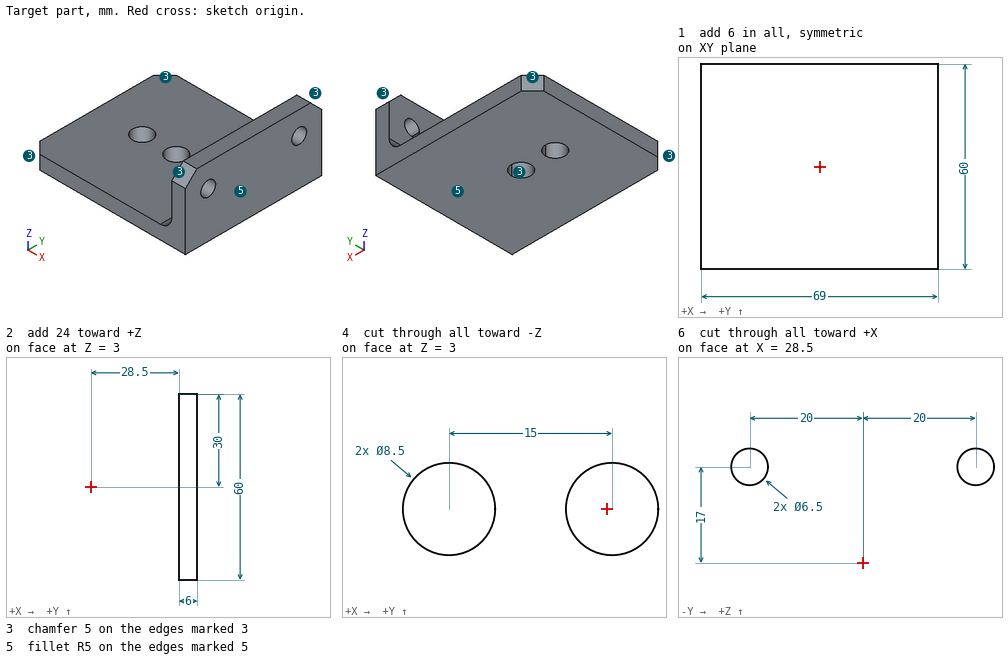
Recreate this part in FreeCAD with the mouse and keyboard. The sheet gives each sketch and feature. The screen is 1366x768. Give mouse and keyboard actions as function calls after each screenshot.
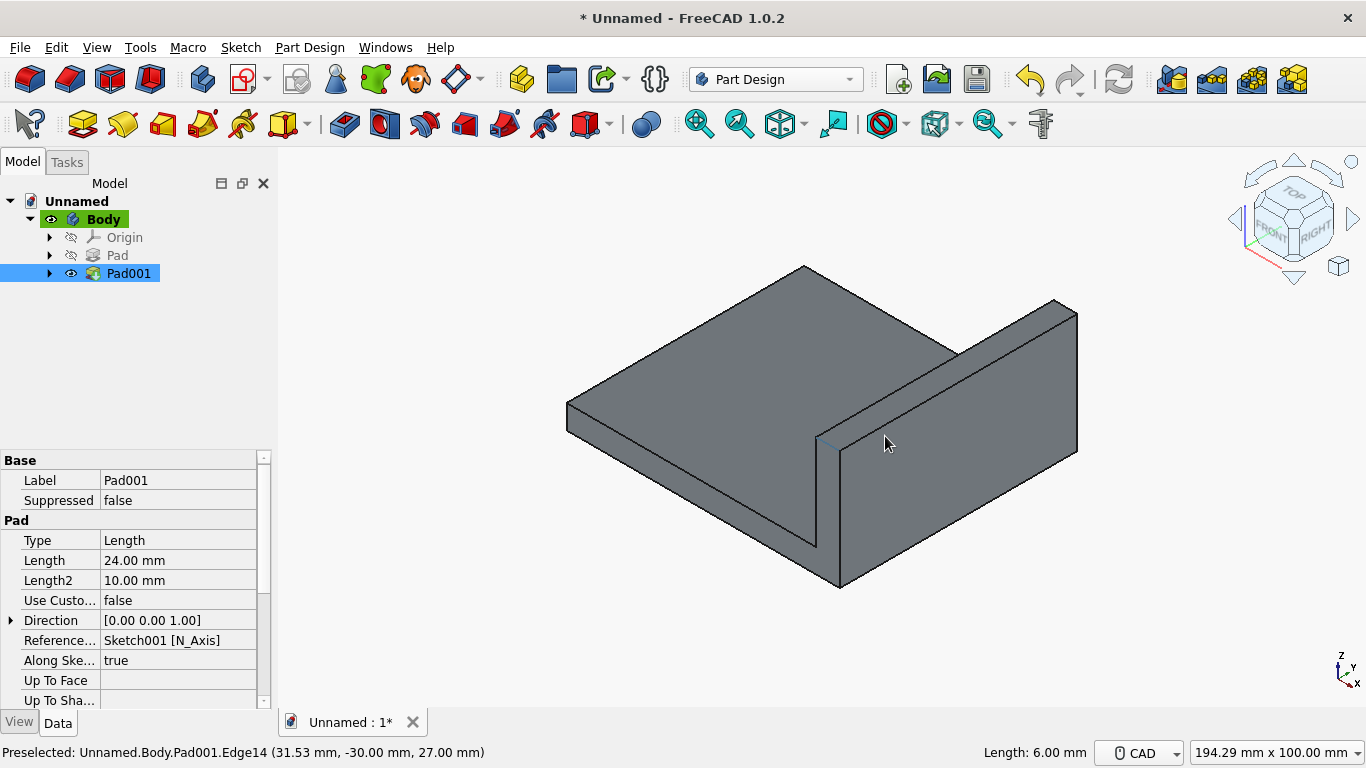
key(2)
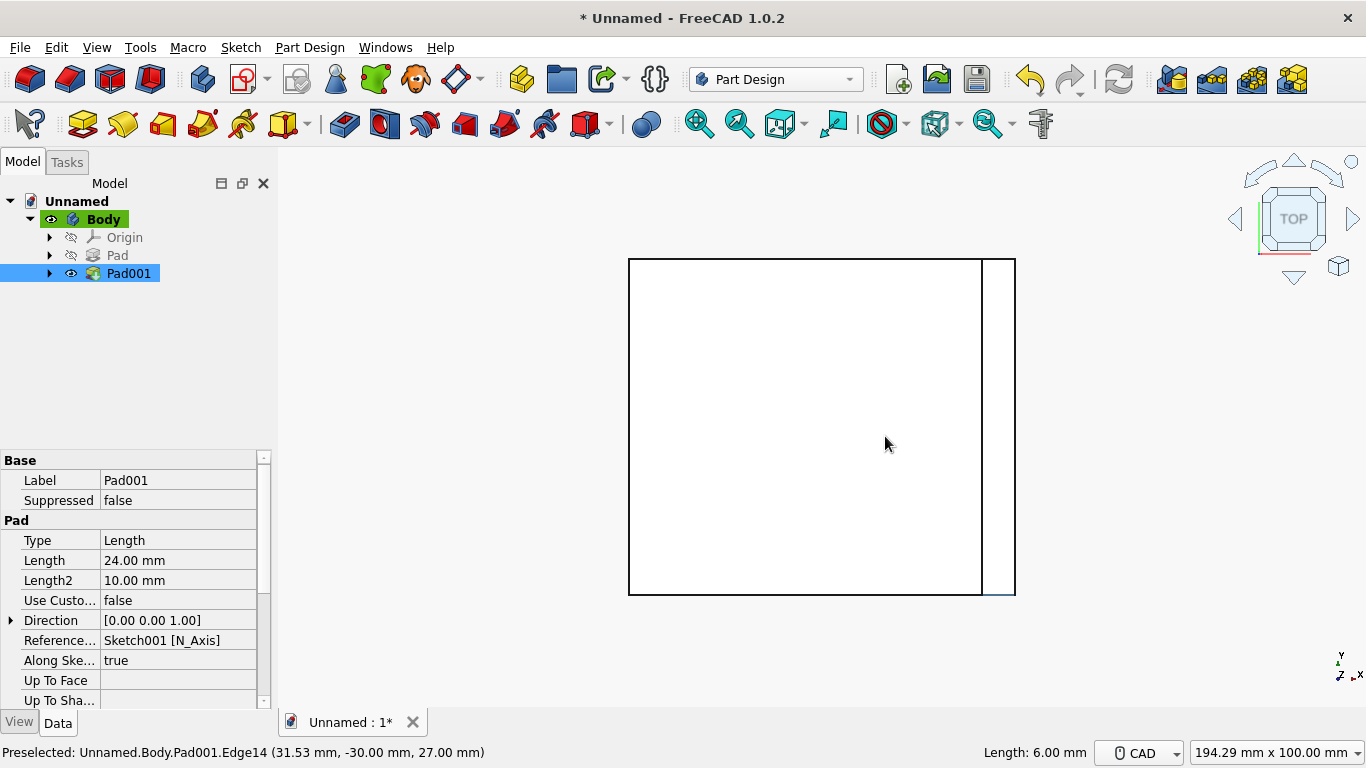
click(998, 258, ctrl)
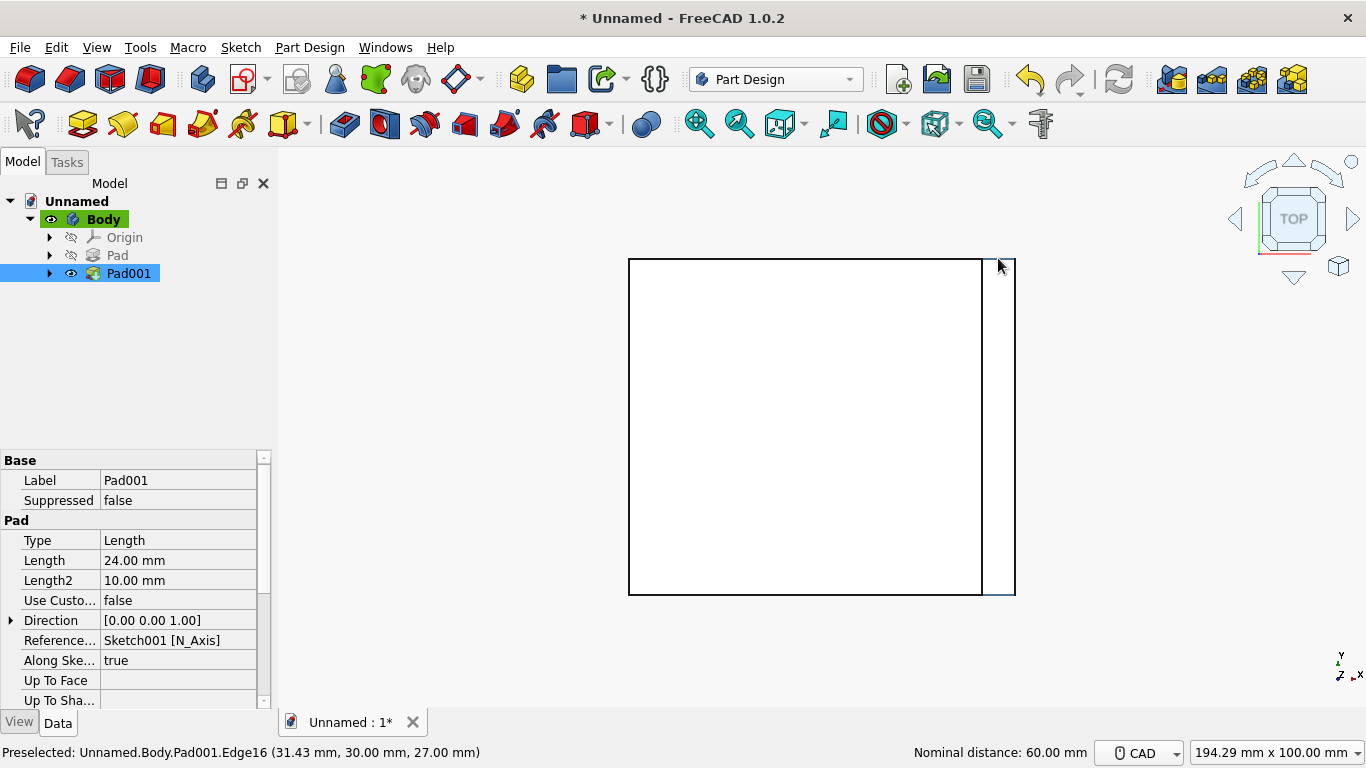
key(1)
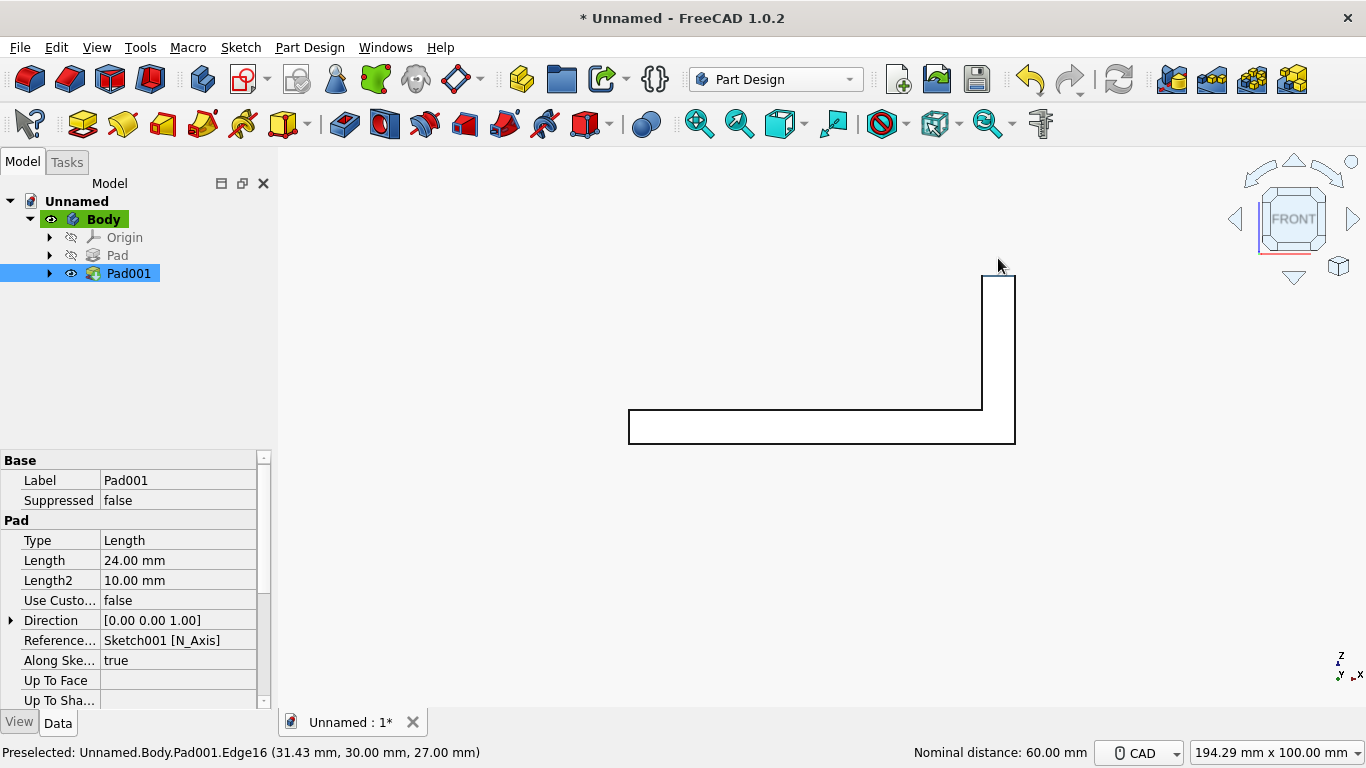
click(700, 124)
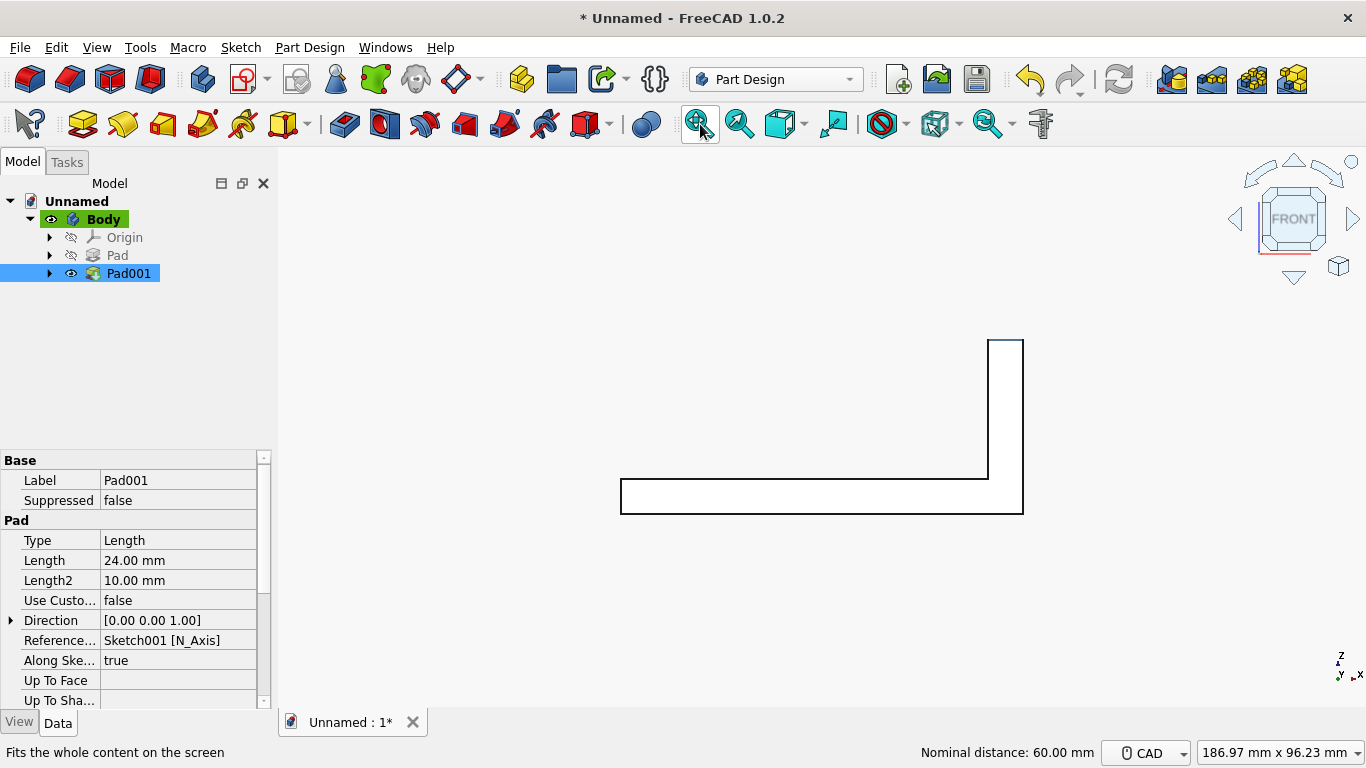
click(621, 496, ctrl)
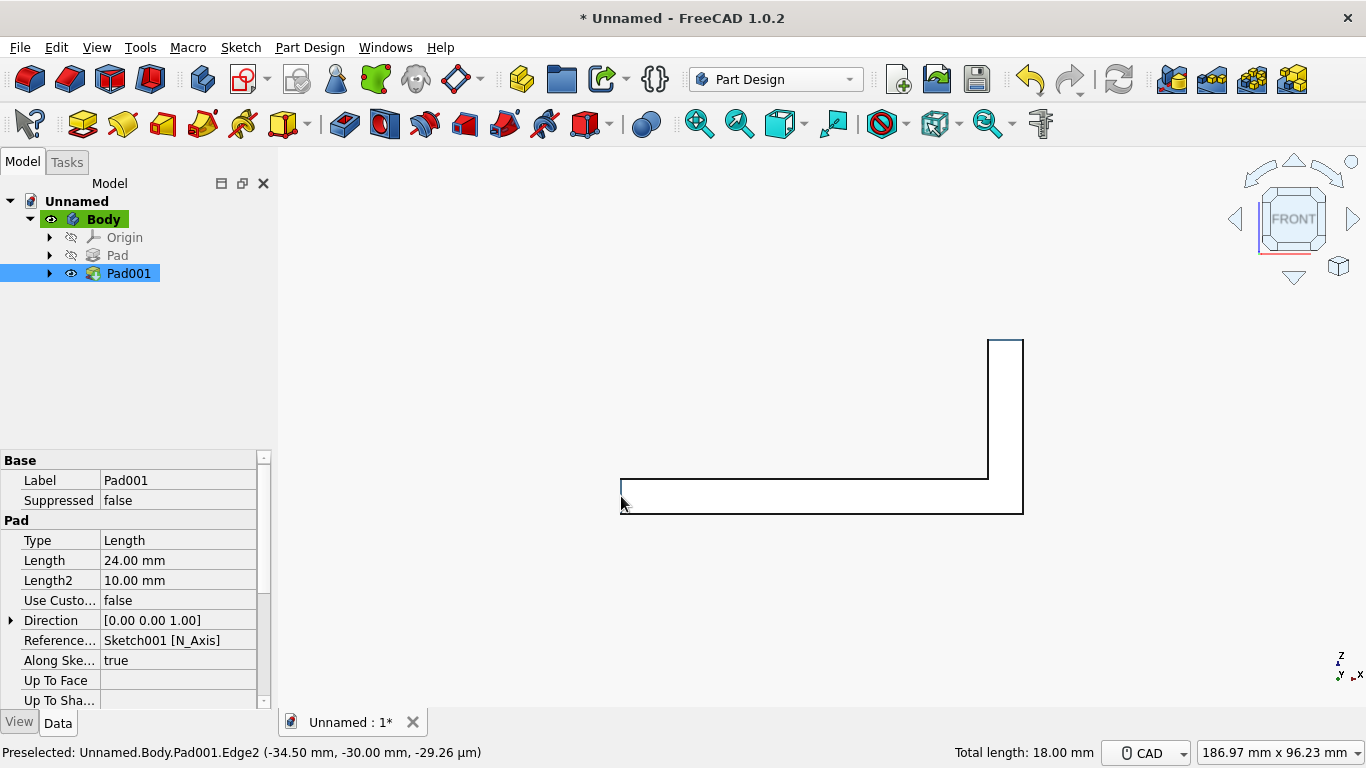
key(3)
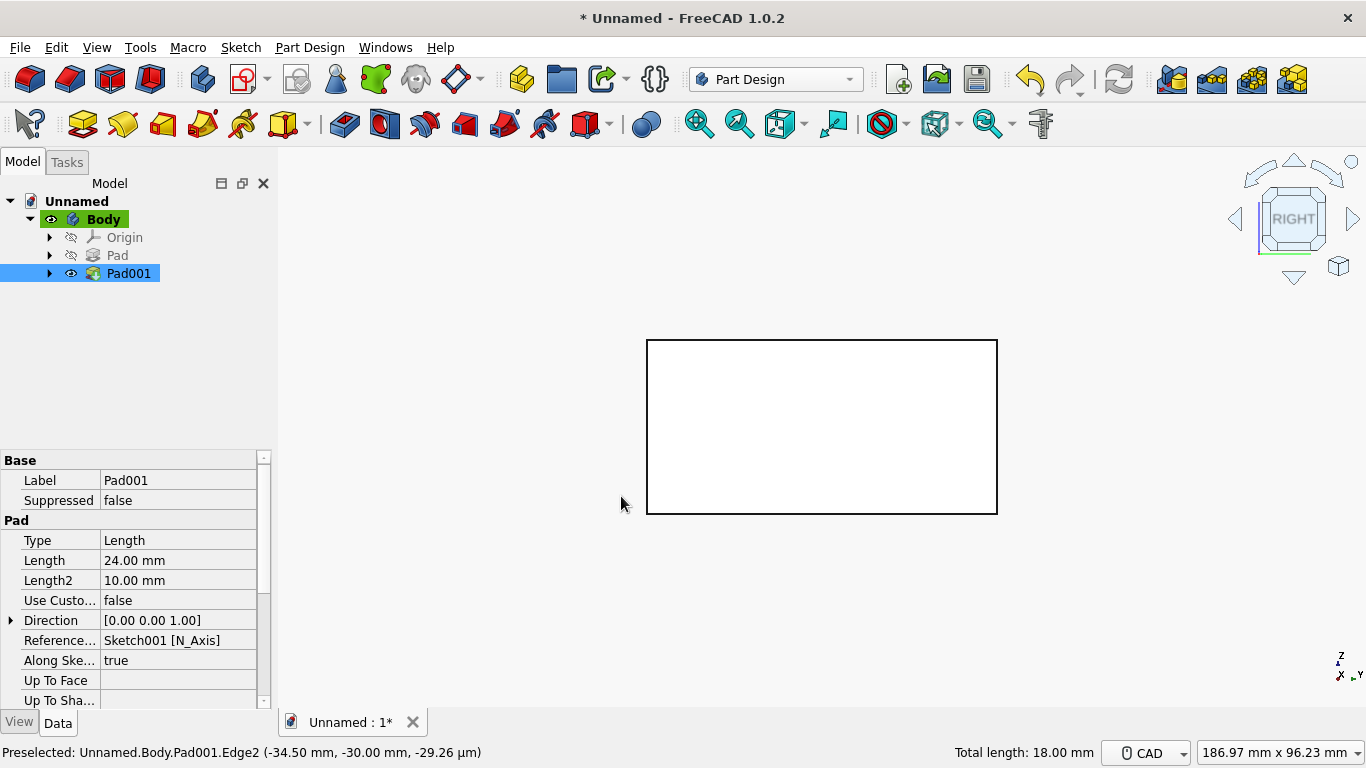
key(v)
key(f)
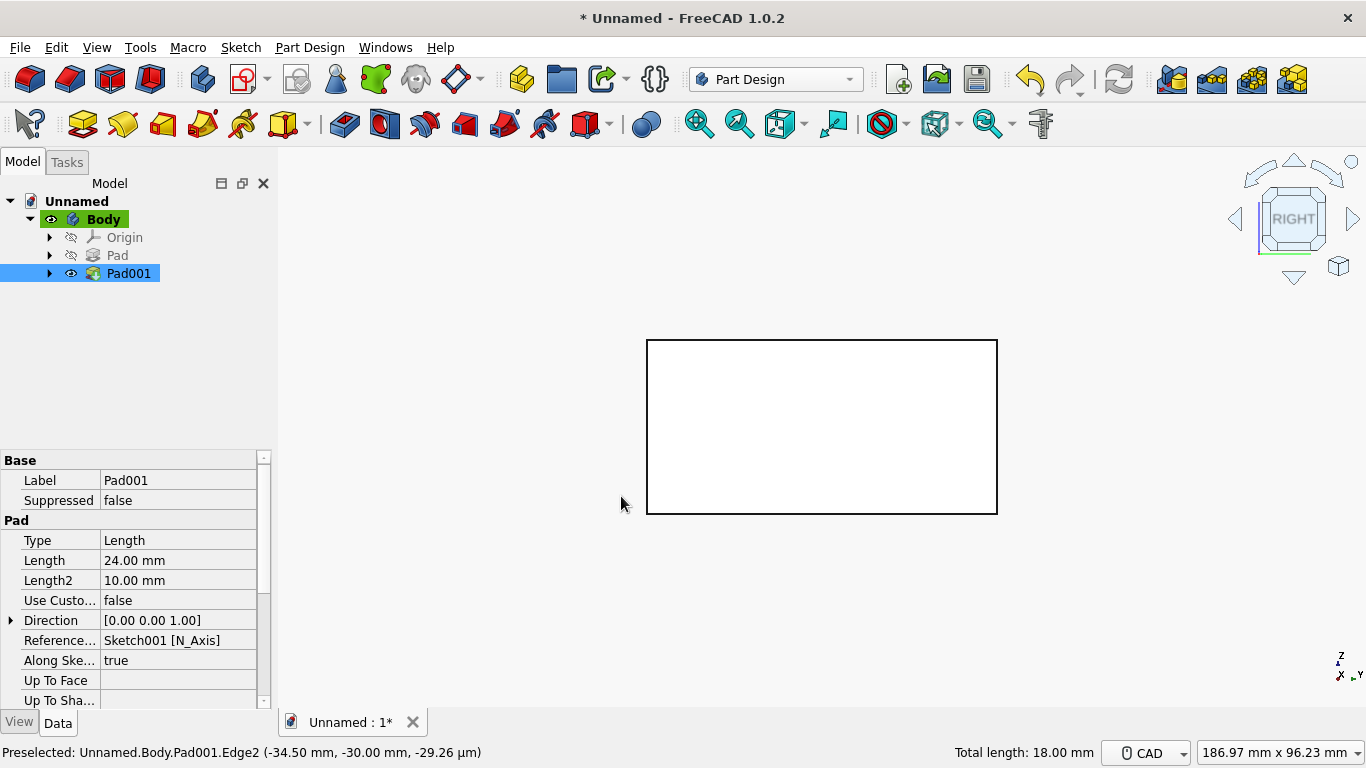
key(5)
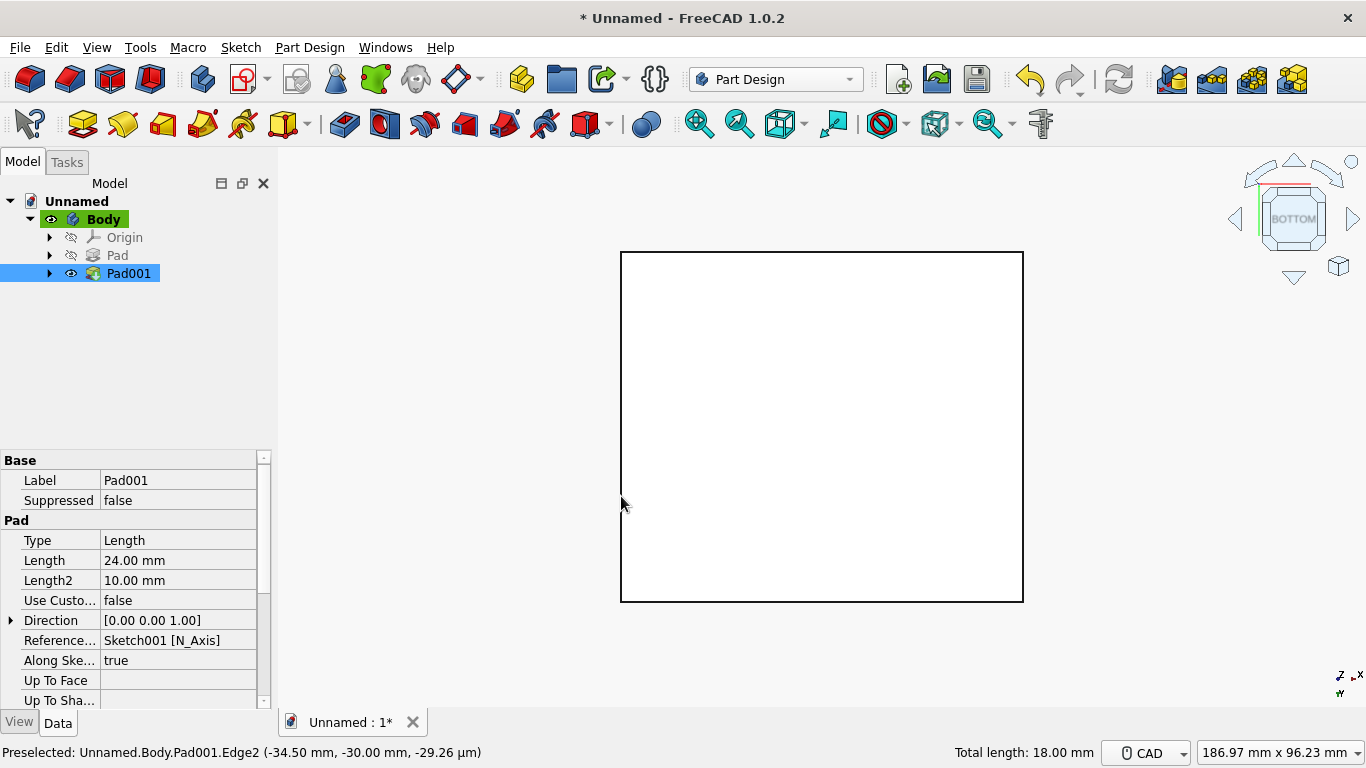
key(4)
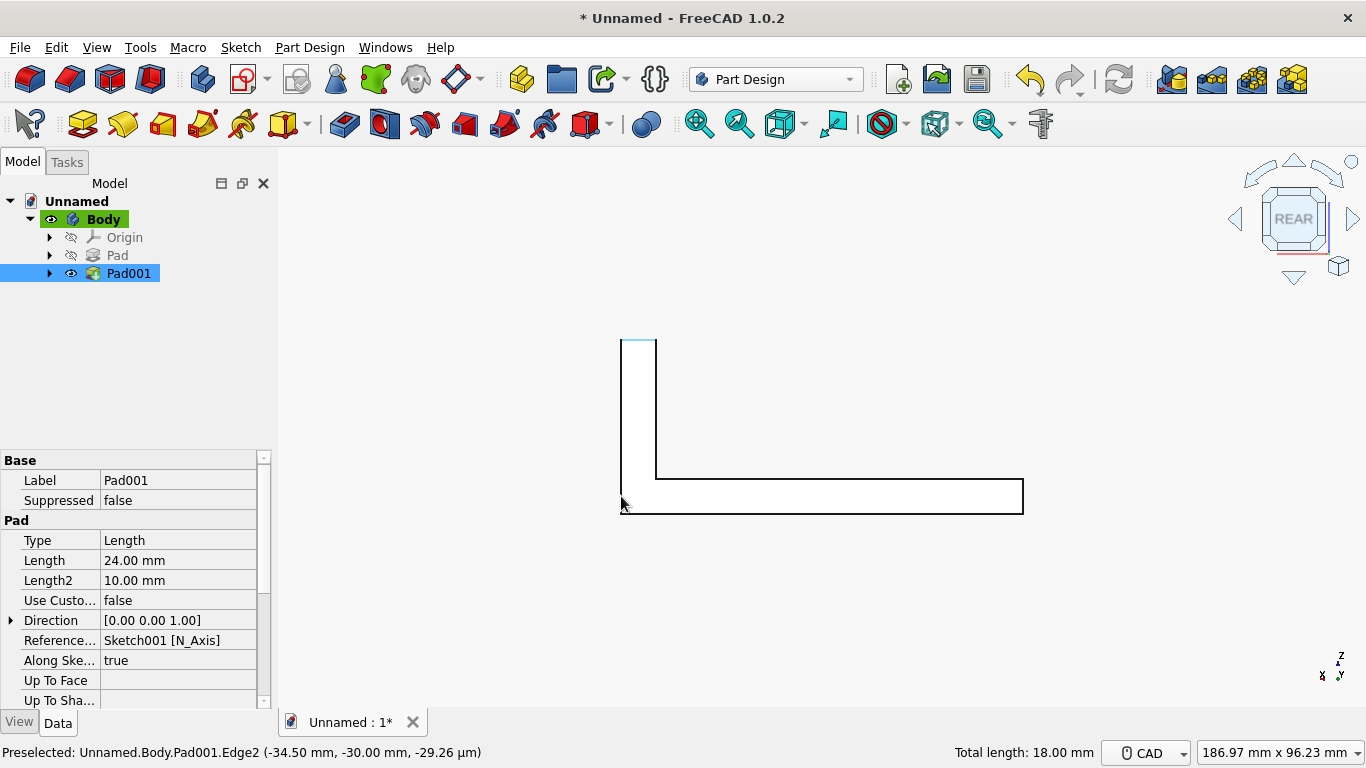
key(v)
key(f)